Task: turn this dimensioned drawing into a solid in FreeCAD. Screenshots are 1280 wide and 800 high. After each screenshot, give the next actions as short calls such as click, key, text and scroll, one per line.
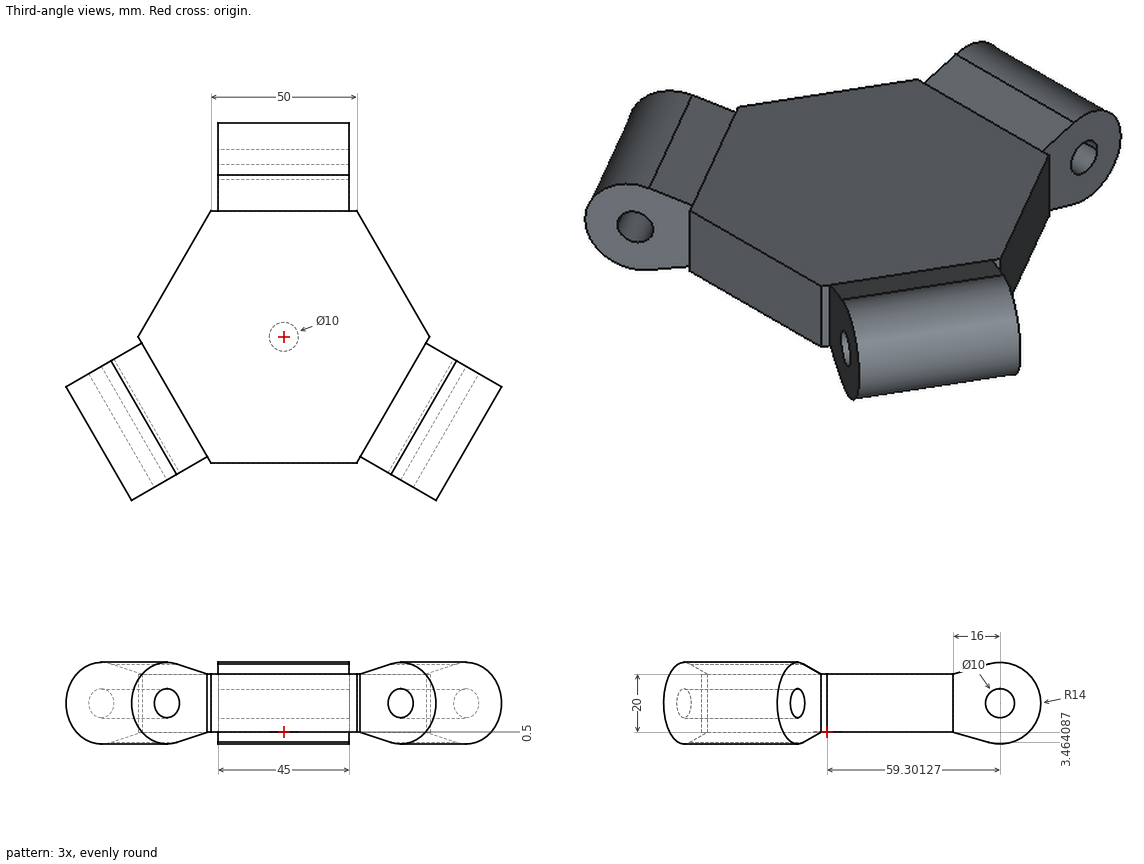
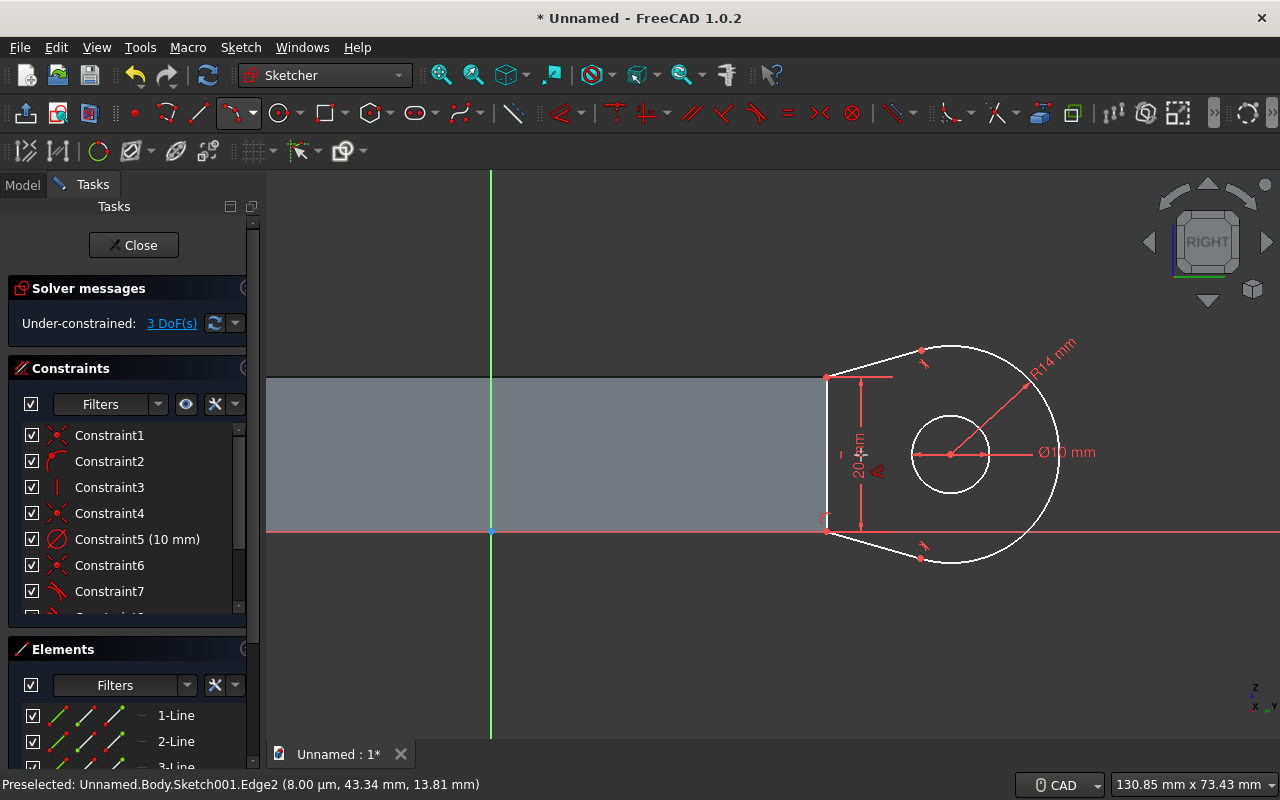
click(827, 377)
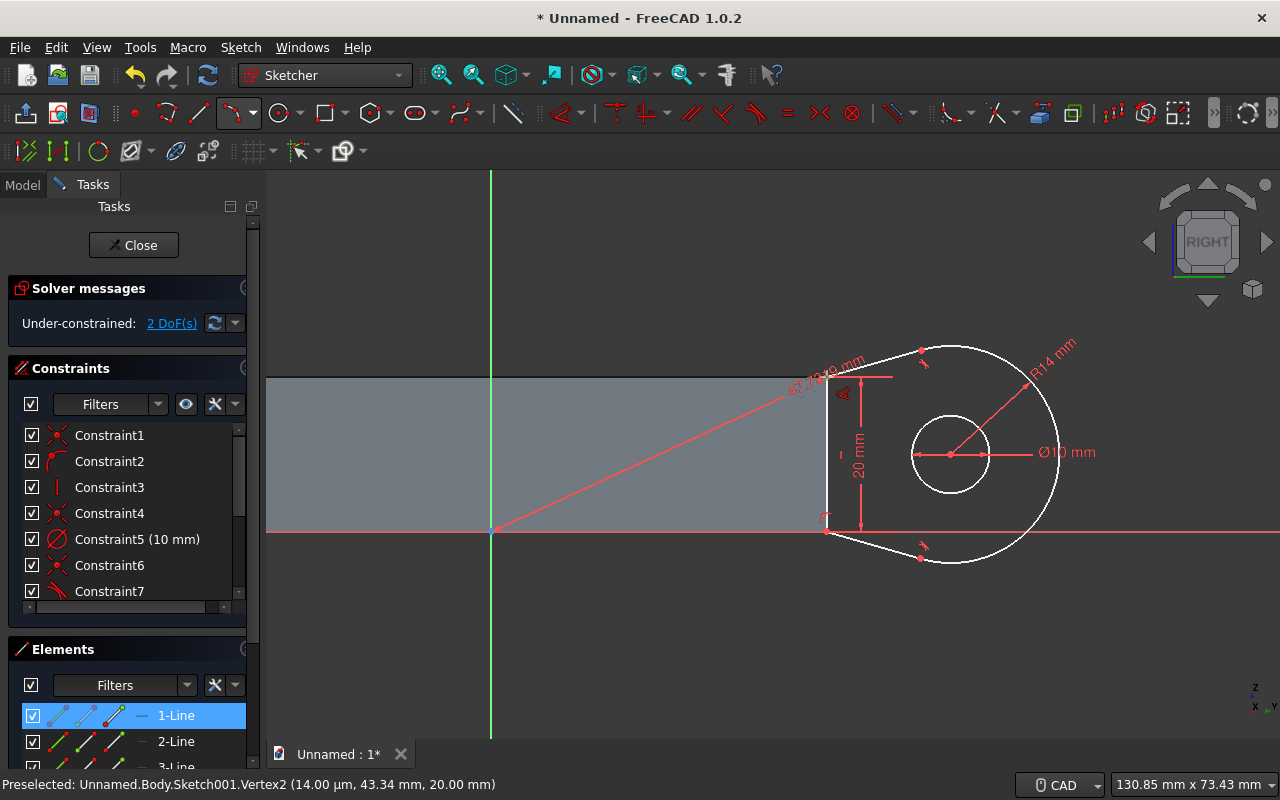
click(951, 455)
click(889, 343)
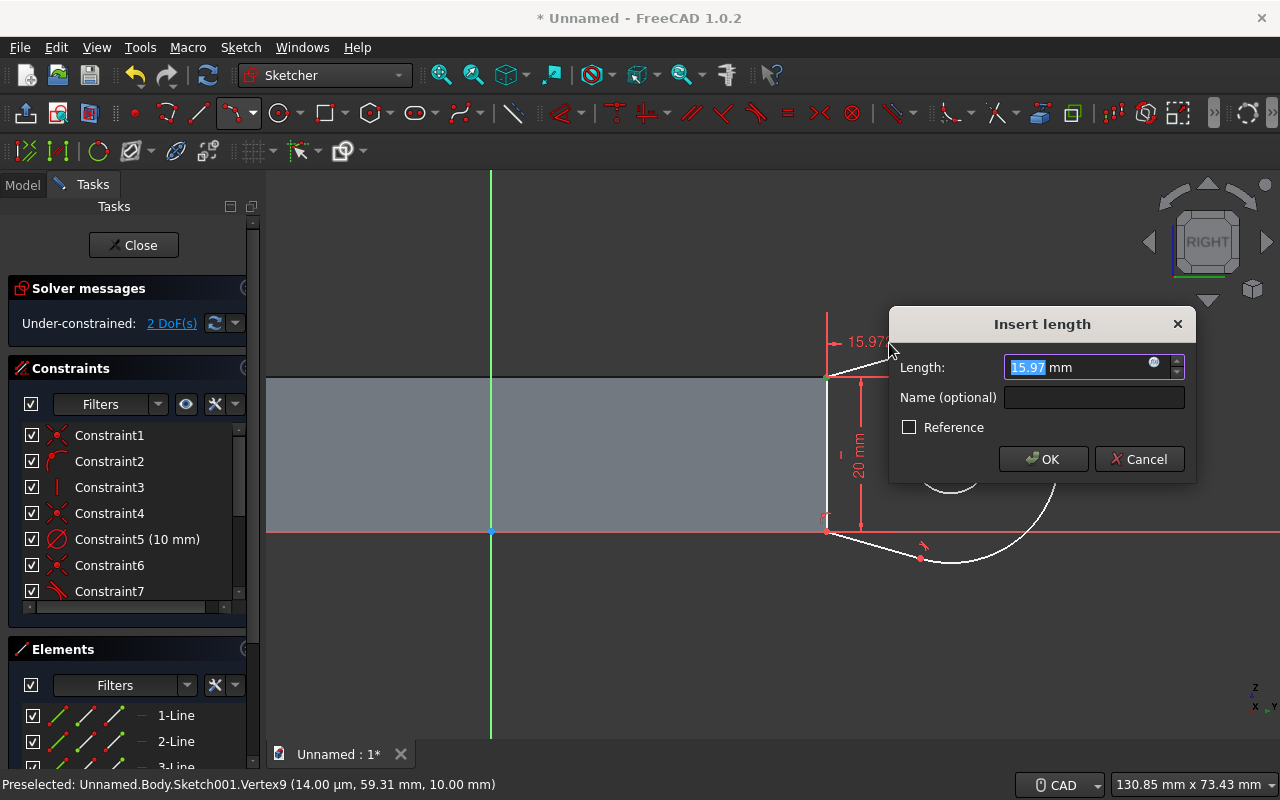
text(16)
key(Return)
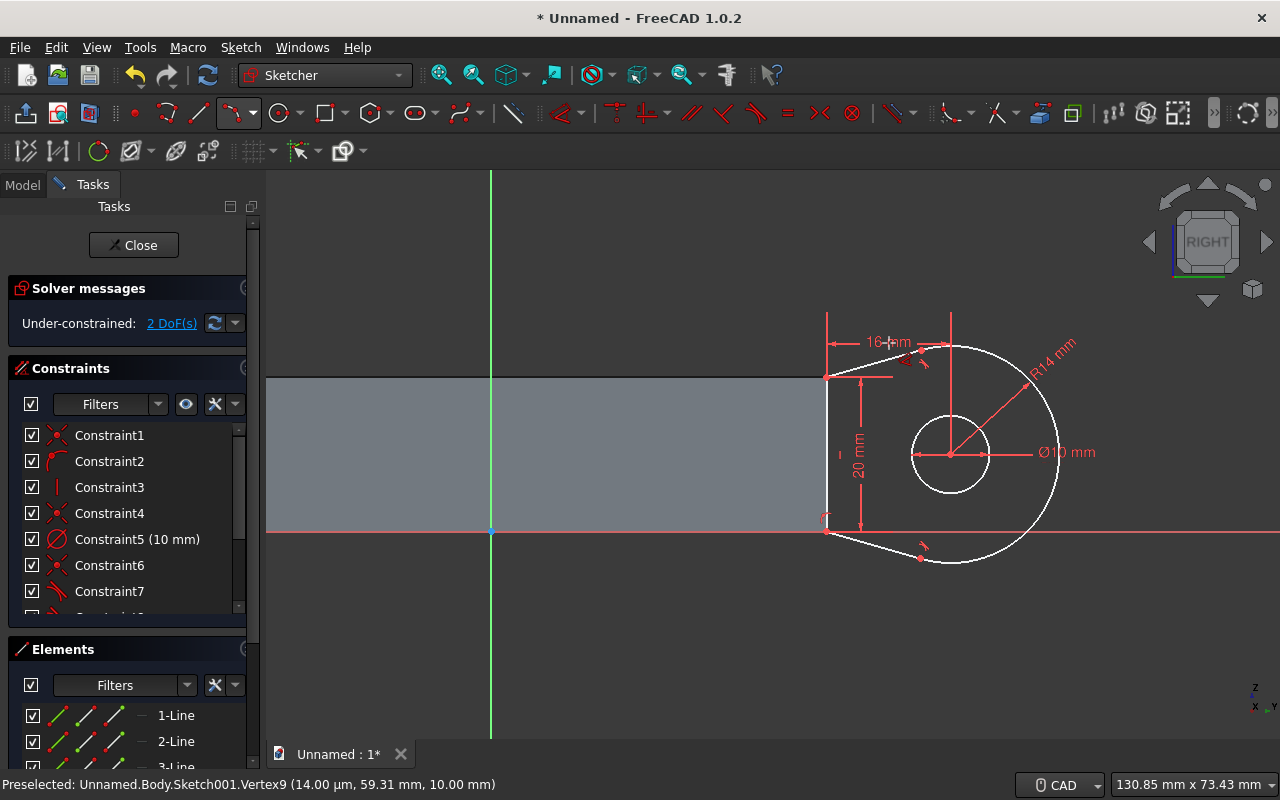
click(951, 455)
click(721, 566)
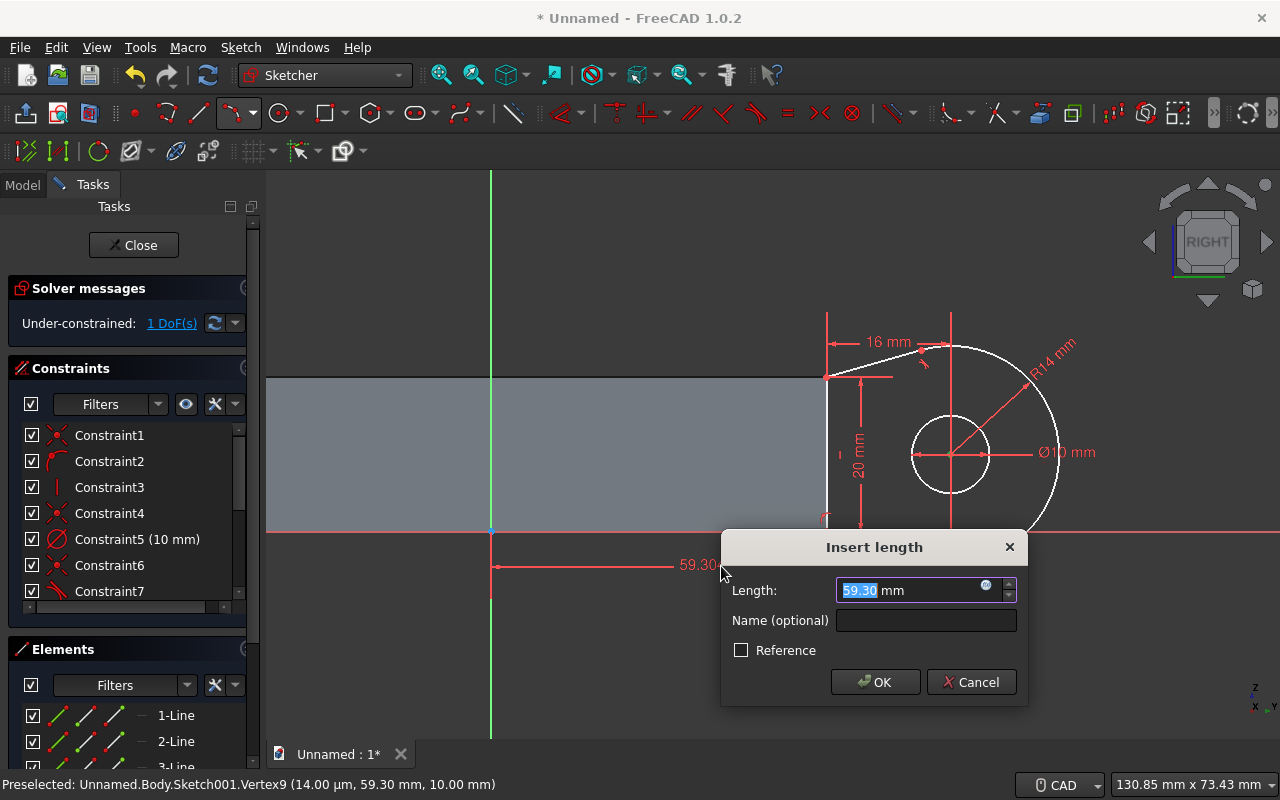
text(59.30127)
key(Return)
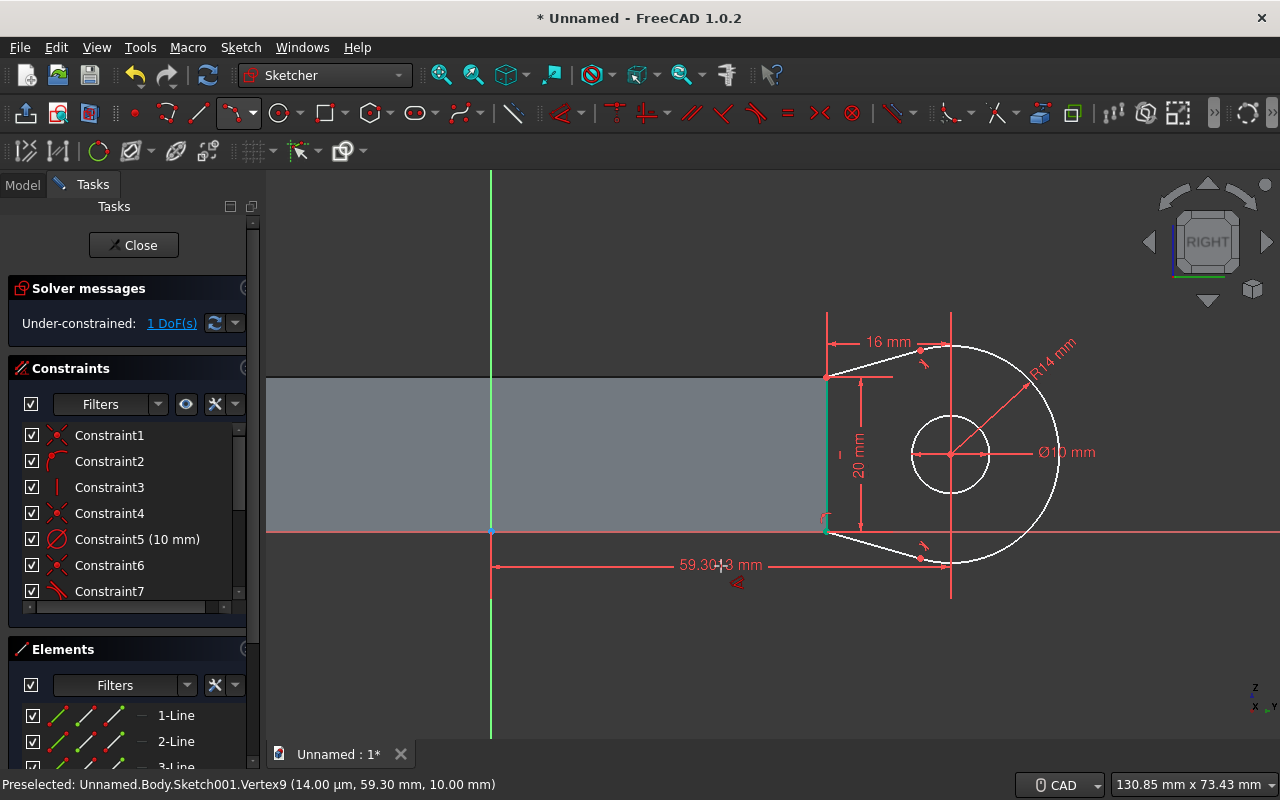
scroll(921, 559, up, 2)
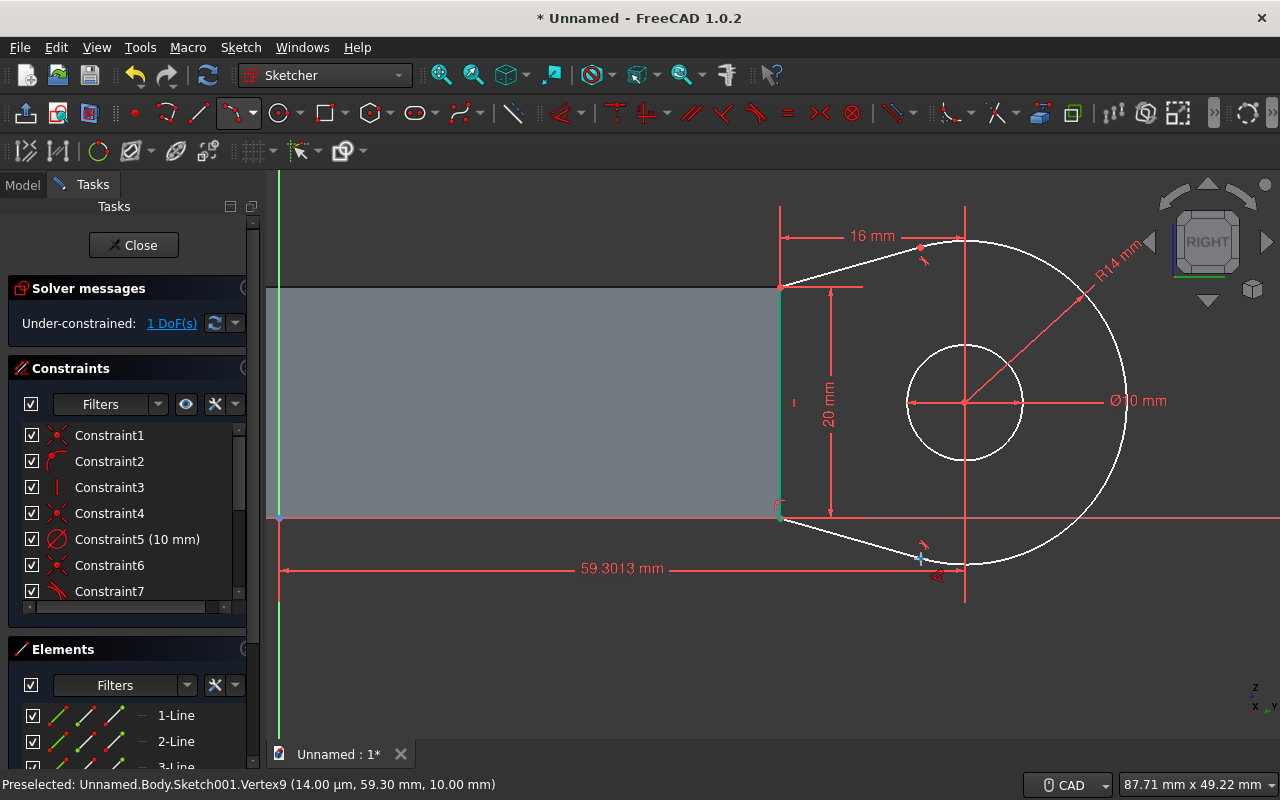
click(921, 558)
click(955, 538)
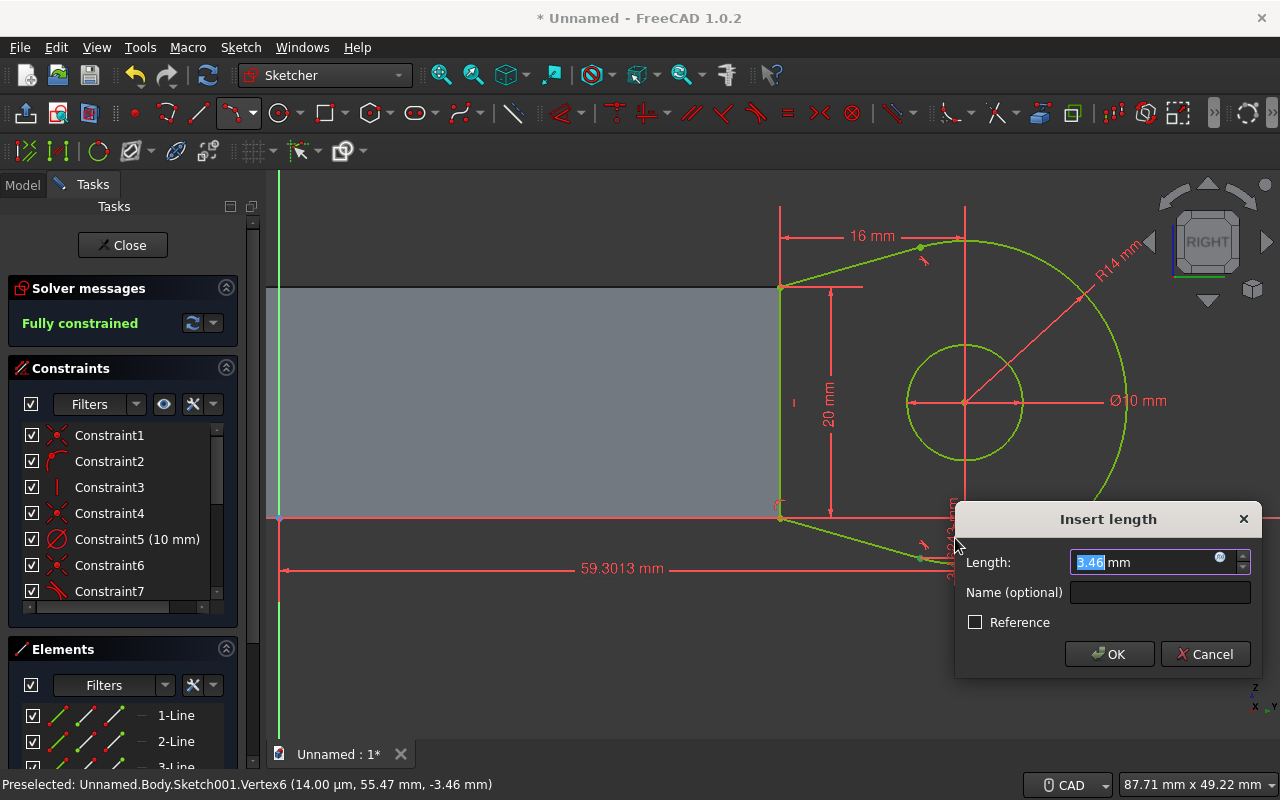
text(3.464087)
key(Return)
key(Escape)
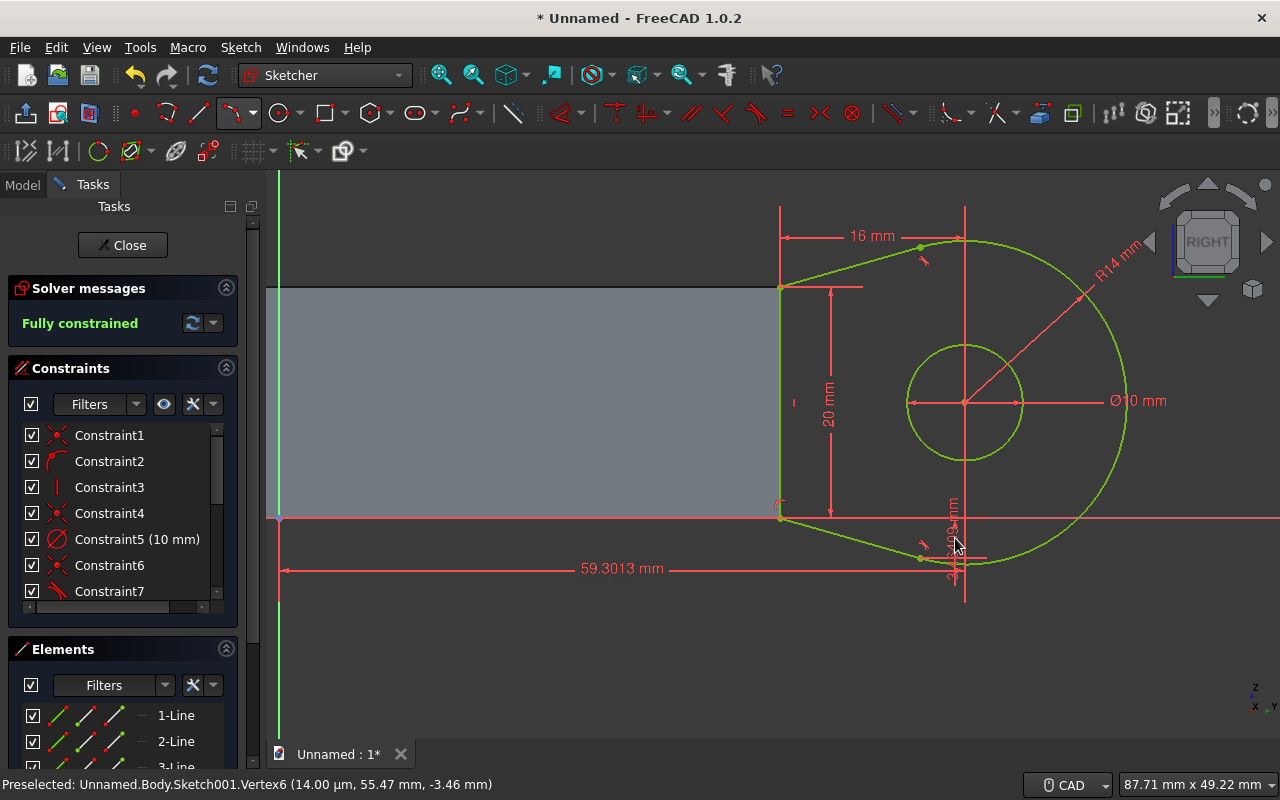
click(123, 245)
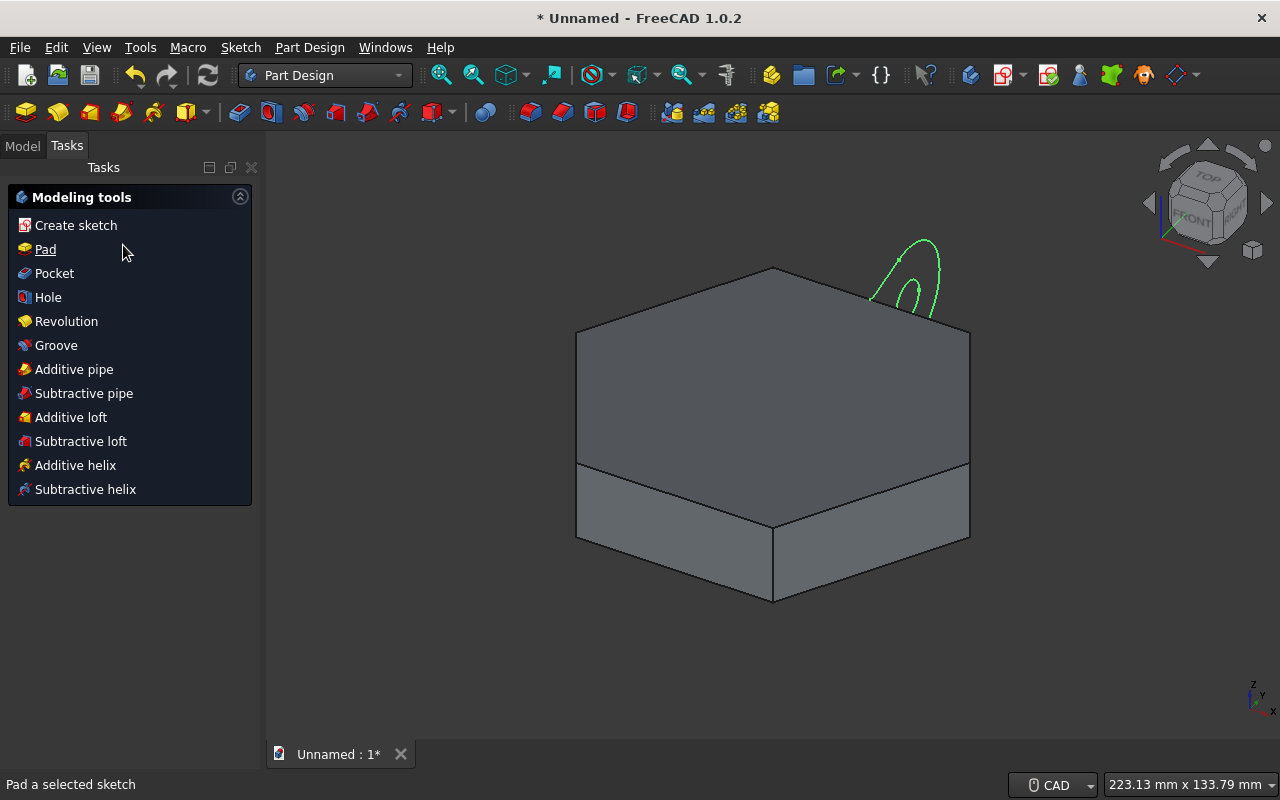
click(26, 112)